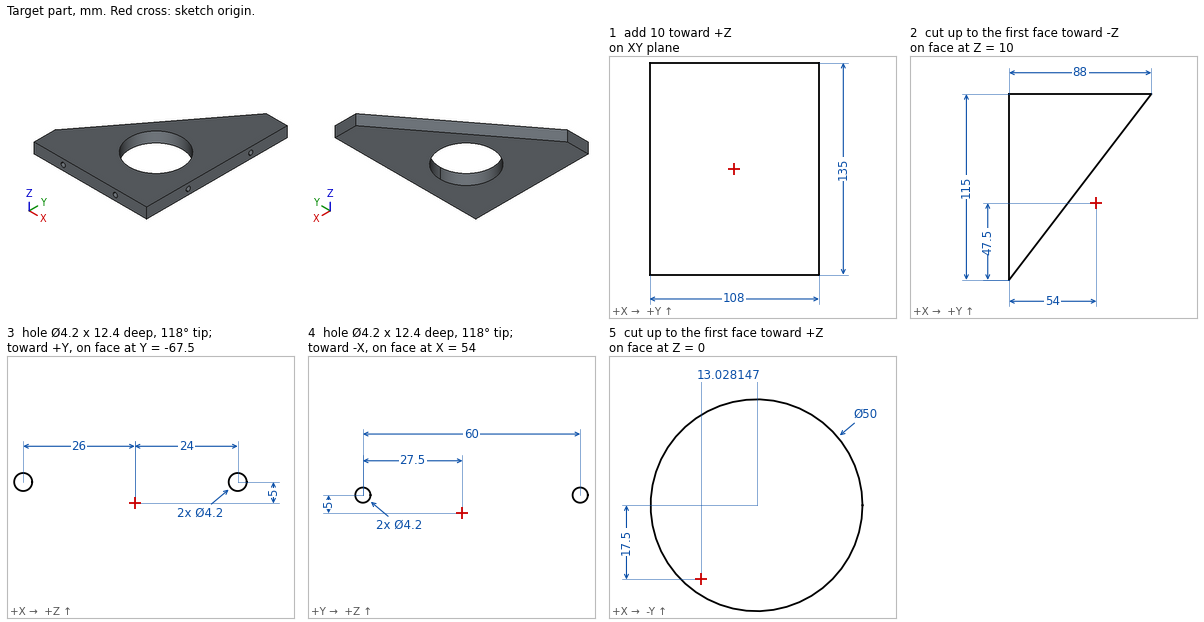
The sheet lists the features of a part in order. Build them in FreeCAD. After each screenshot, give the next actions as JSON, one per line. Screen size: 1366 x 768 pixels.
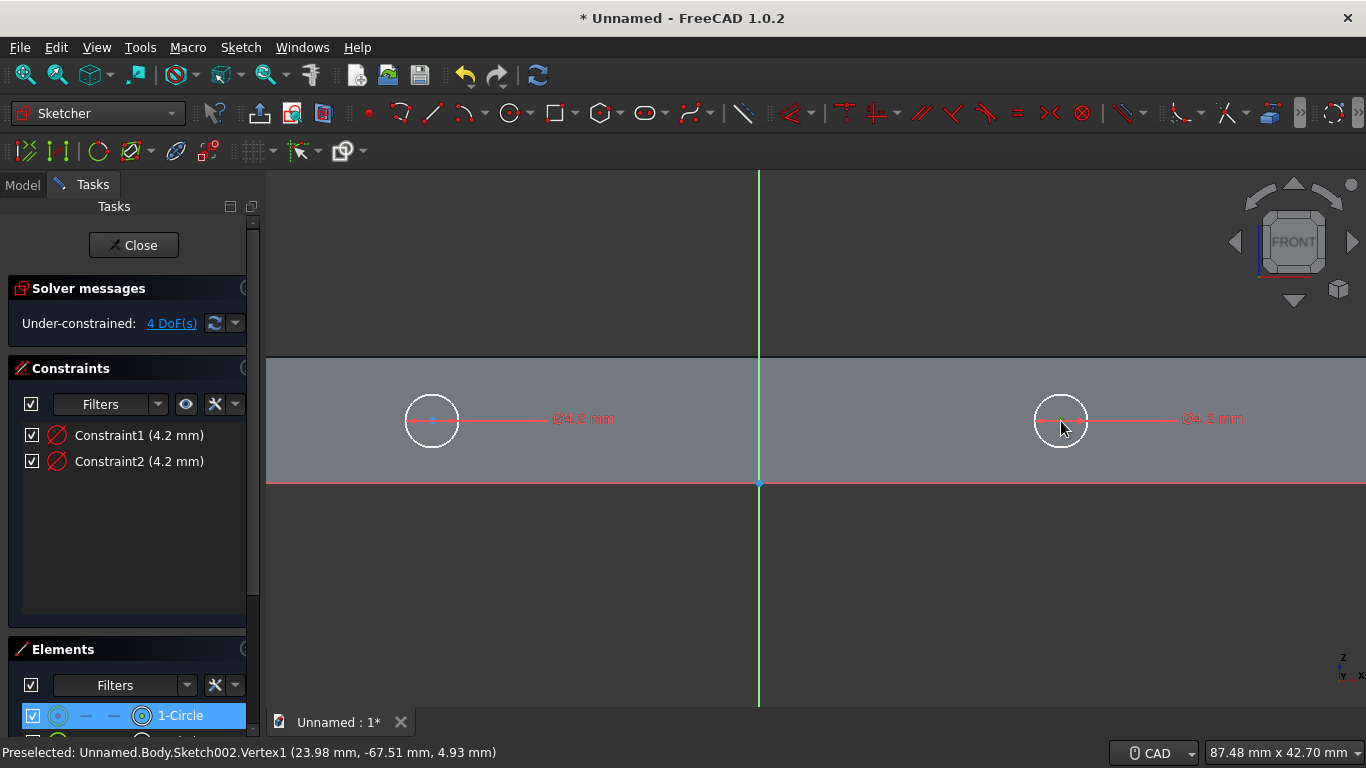
{"action": "left_click", "coordinate": [432, 421]}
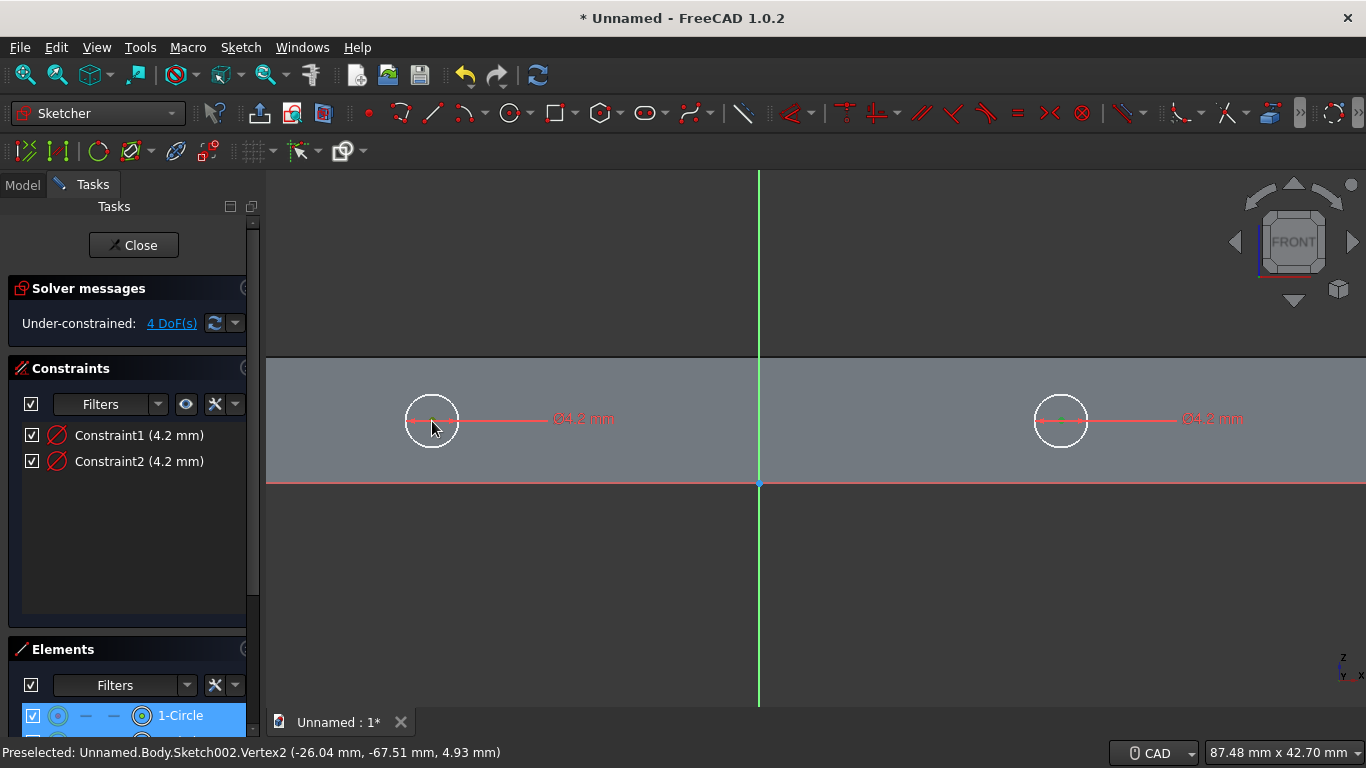
{"action": "key", "text": "h"}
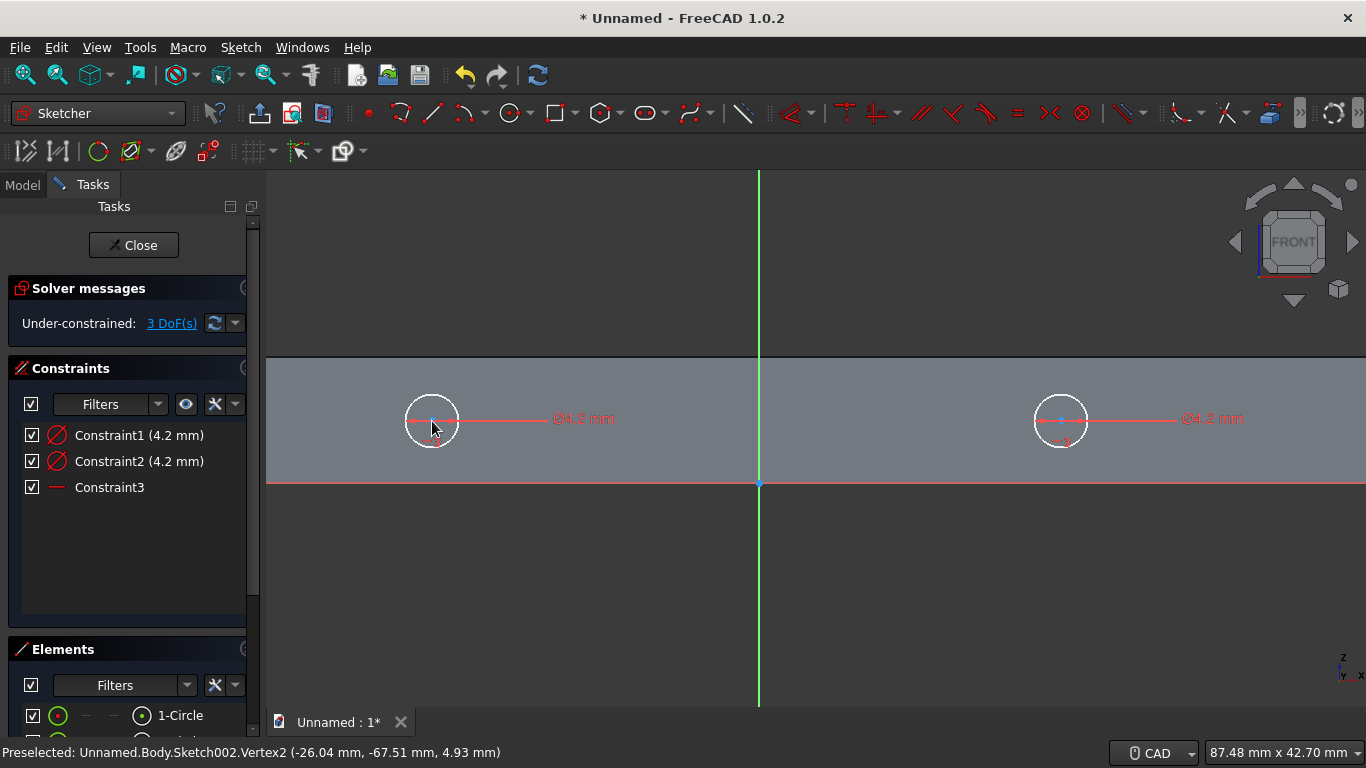
{"action": "key", "text": "d"}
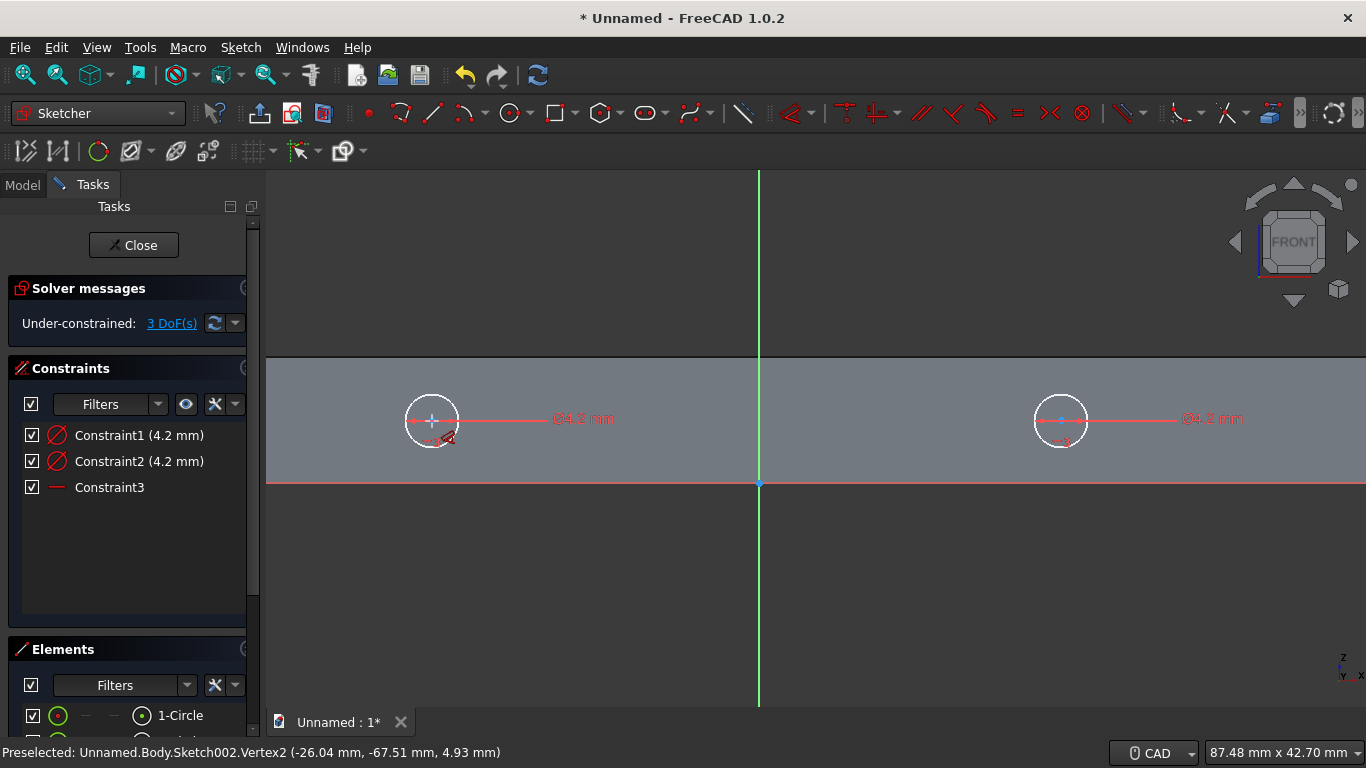
{"action": "left_click", "coordinate": [1061, 421]}
{"action": "left_click", "coordinate": [1095, 452]}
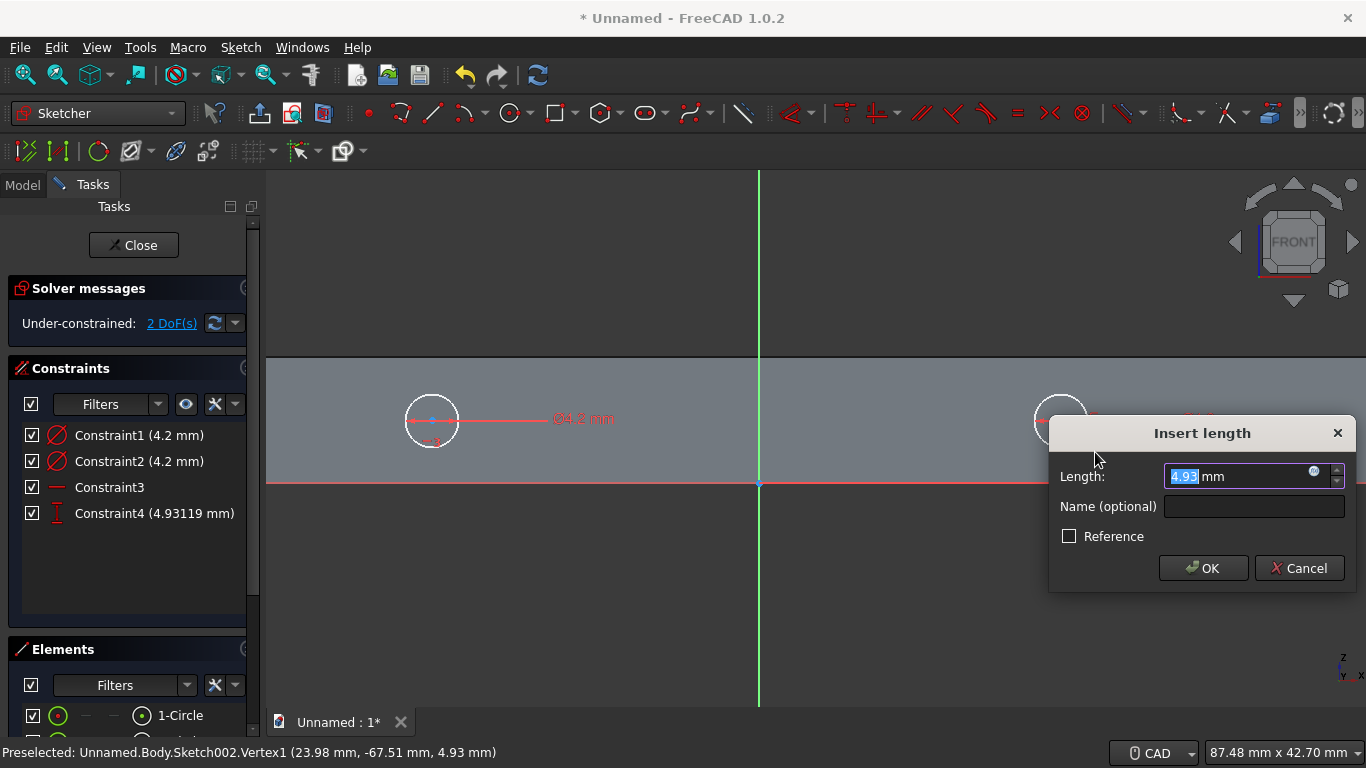
{"action": "type", "text": "5"}
{"action": "key", "text": "Return"}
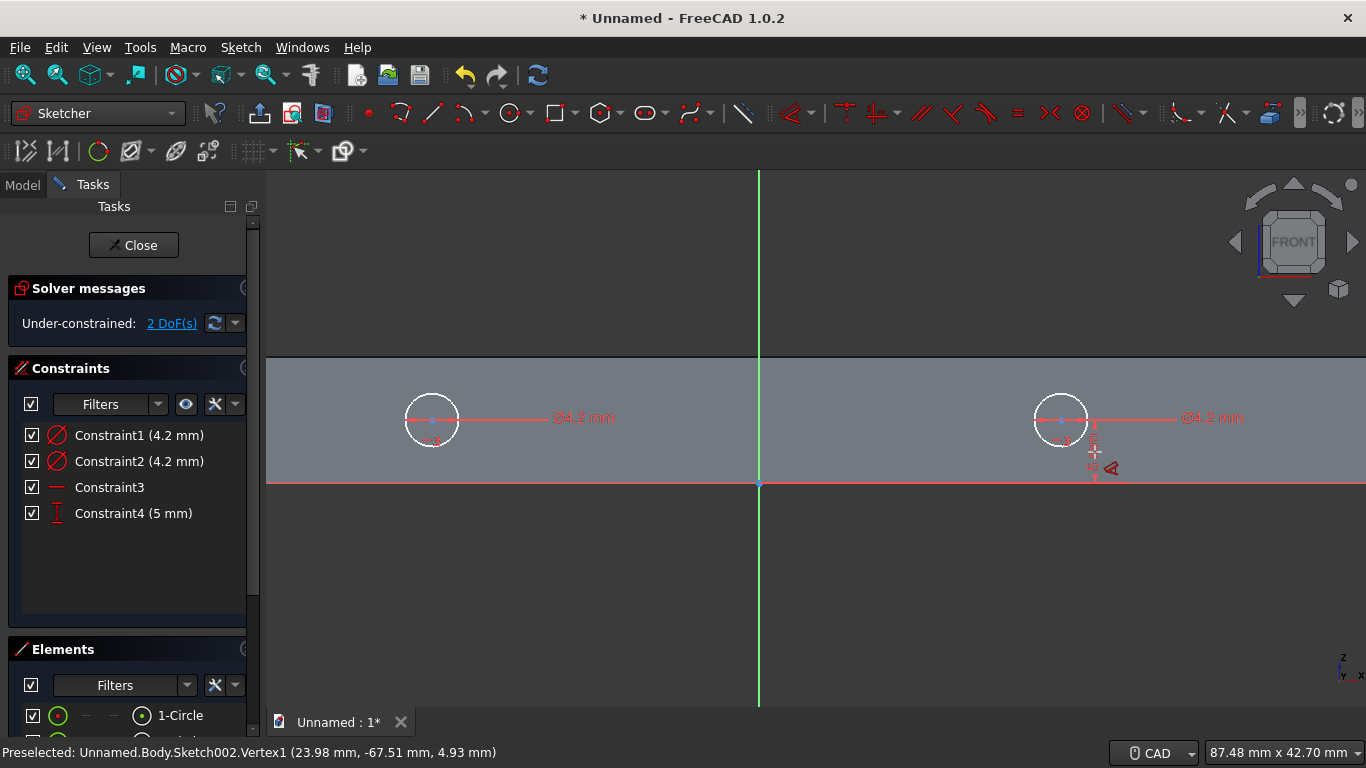
{"action": "left_click", "coordinate": [1061, 420]}
{"action": "left_click", "coordinate": [910, 517]}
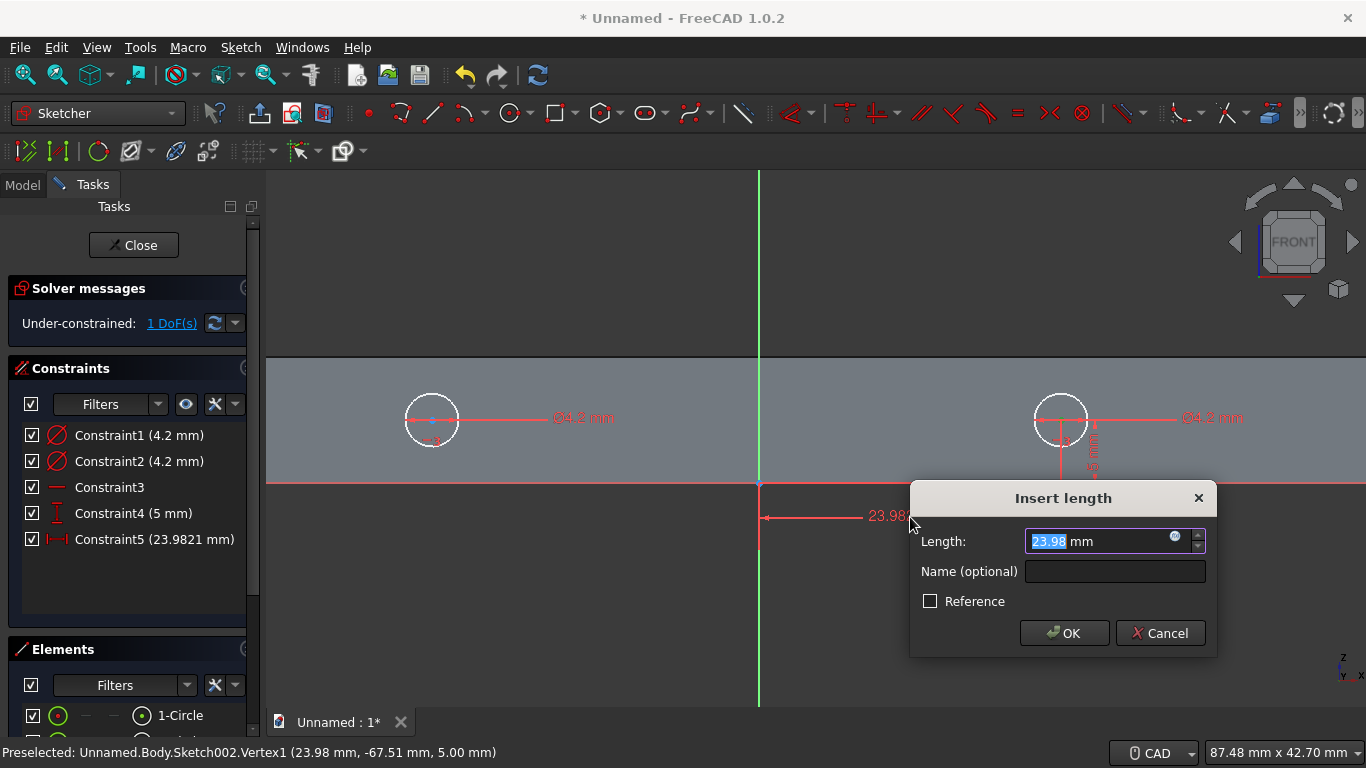
{"action": "type", "text": "24"}
{"action": "key", "text": "Return"}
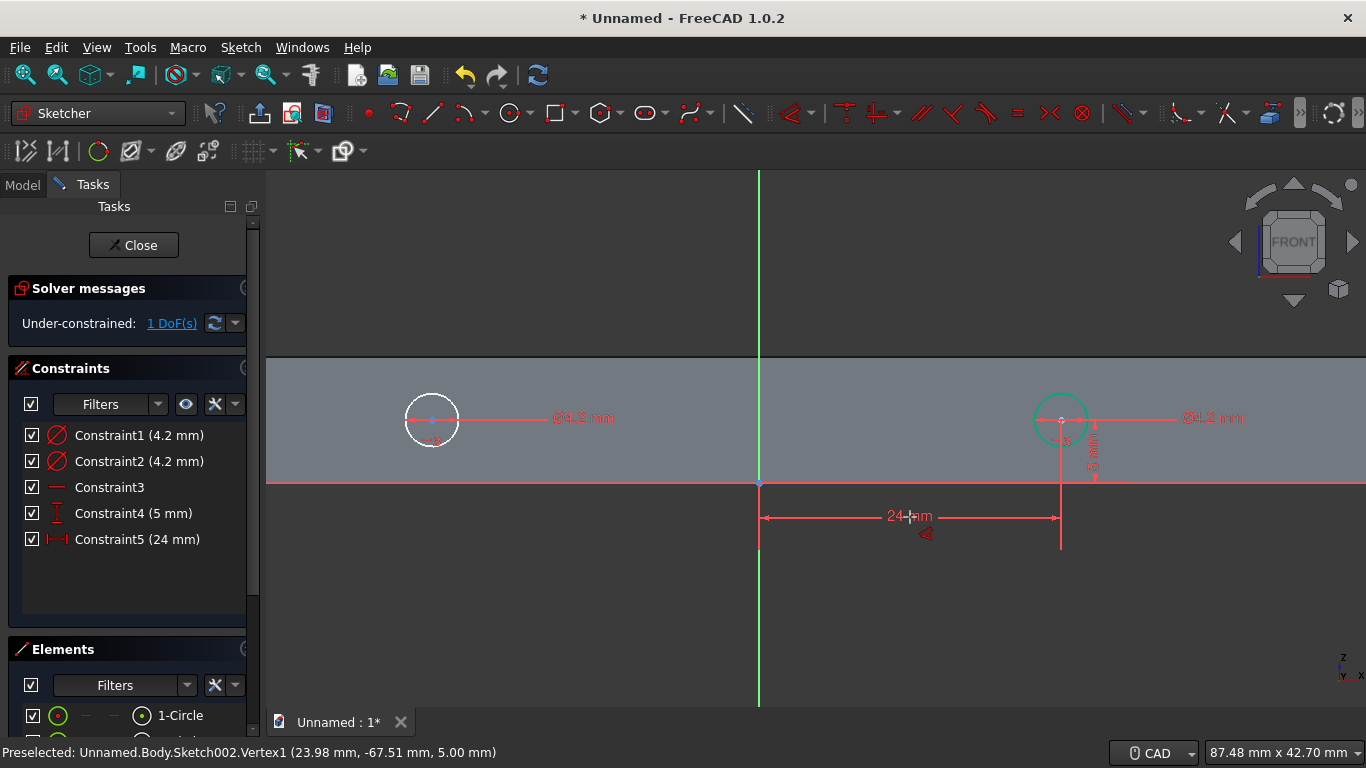
{"action": "left_click", "coordinate": [432, 420]}
{"action": "left_click", "coordinate": [596, 517]}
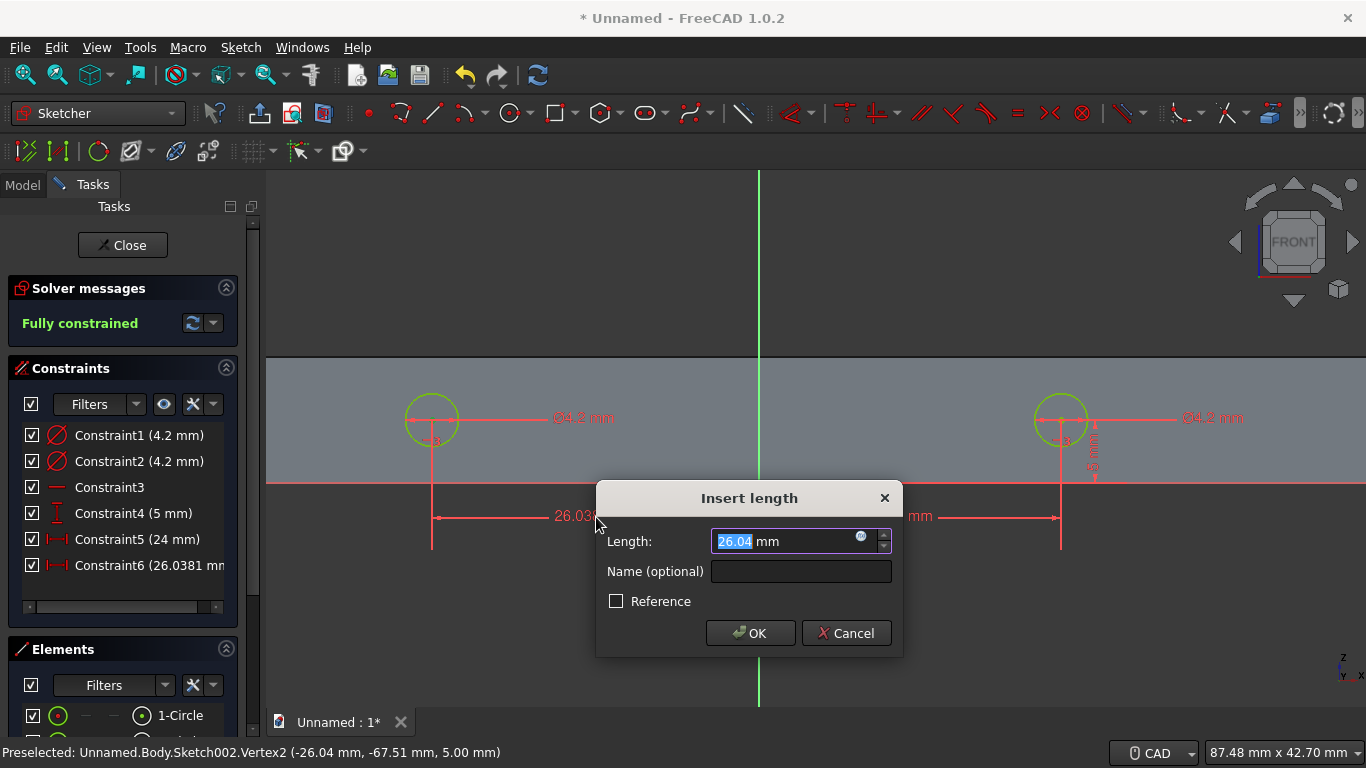
{"action": "type", "text": "26"}
{"action": "key", "text": "Return"}
{"action": "key", "text": "Escape"}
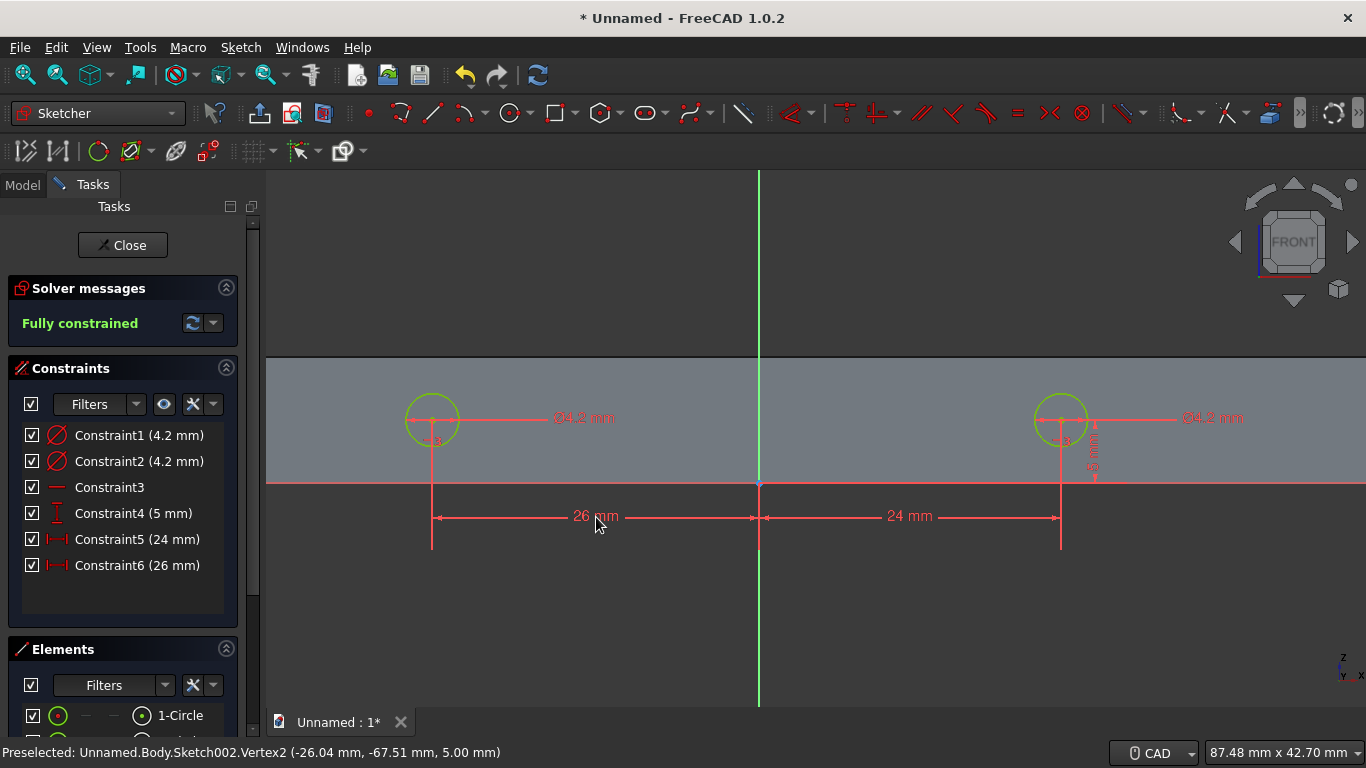
{"action": "left_click", "coordinate": [123, 245]}